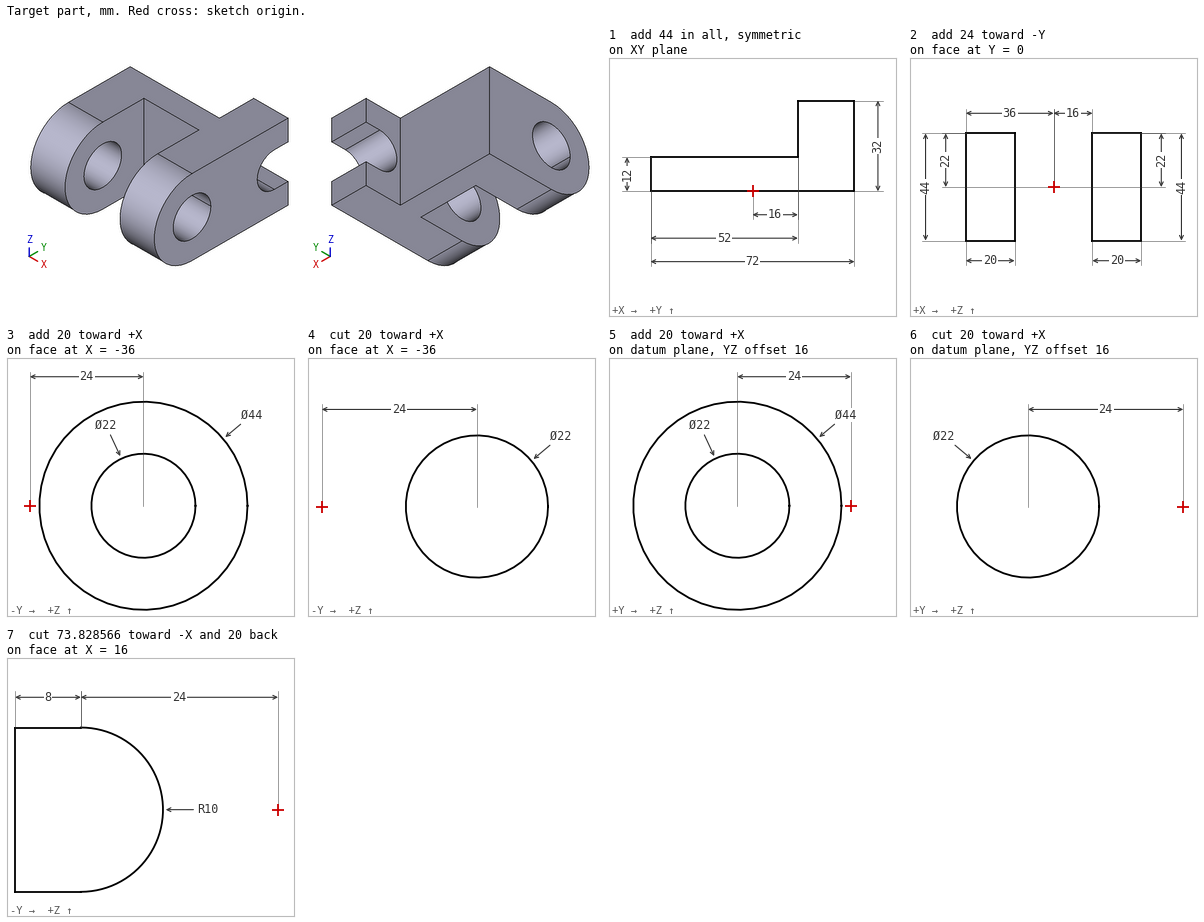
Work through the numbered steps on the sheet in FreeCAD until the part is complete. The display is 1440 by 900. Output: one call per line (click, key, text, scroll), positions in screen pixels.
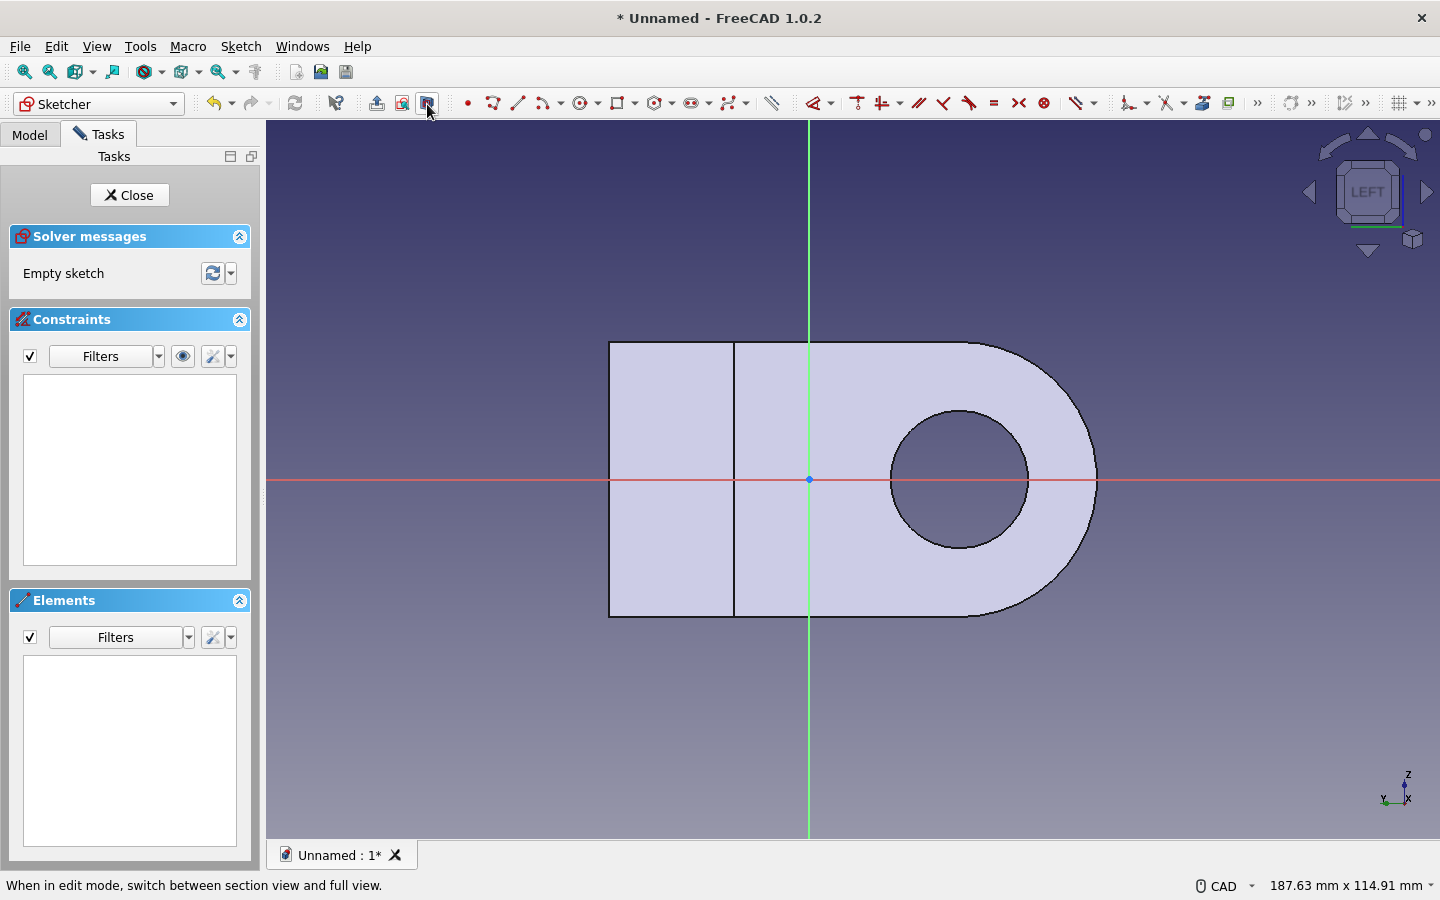
scroll(677, 480, up, 6)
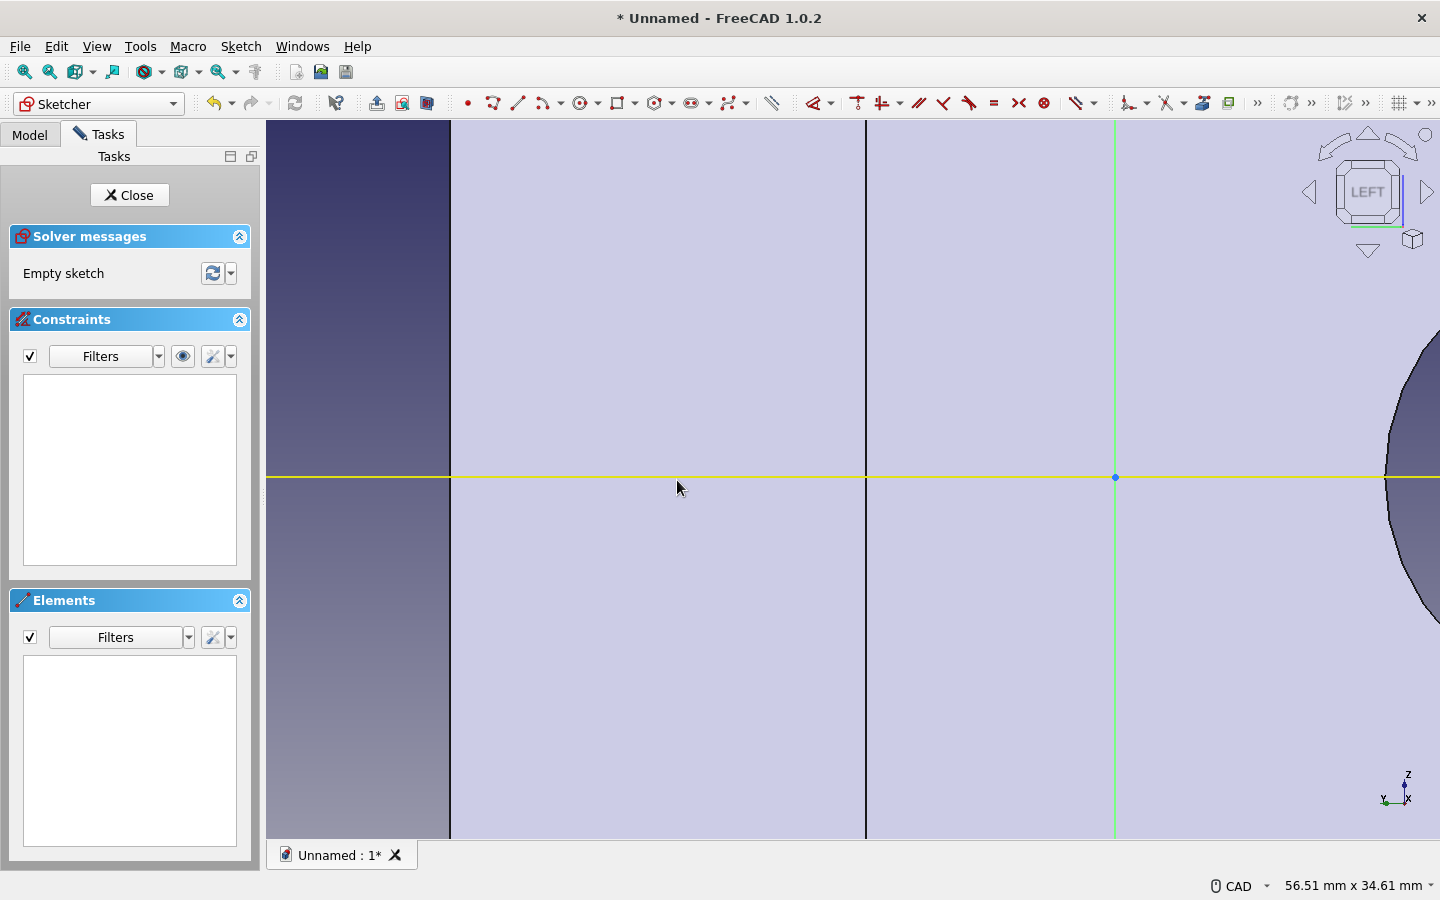
click(493, 104)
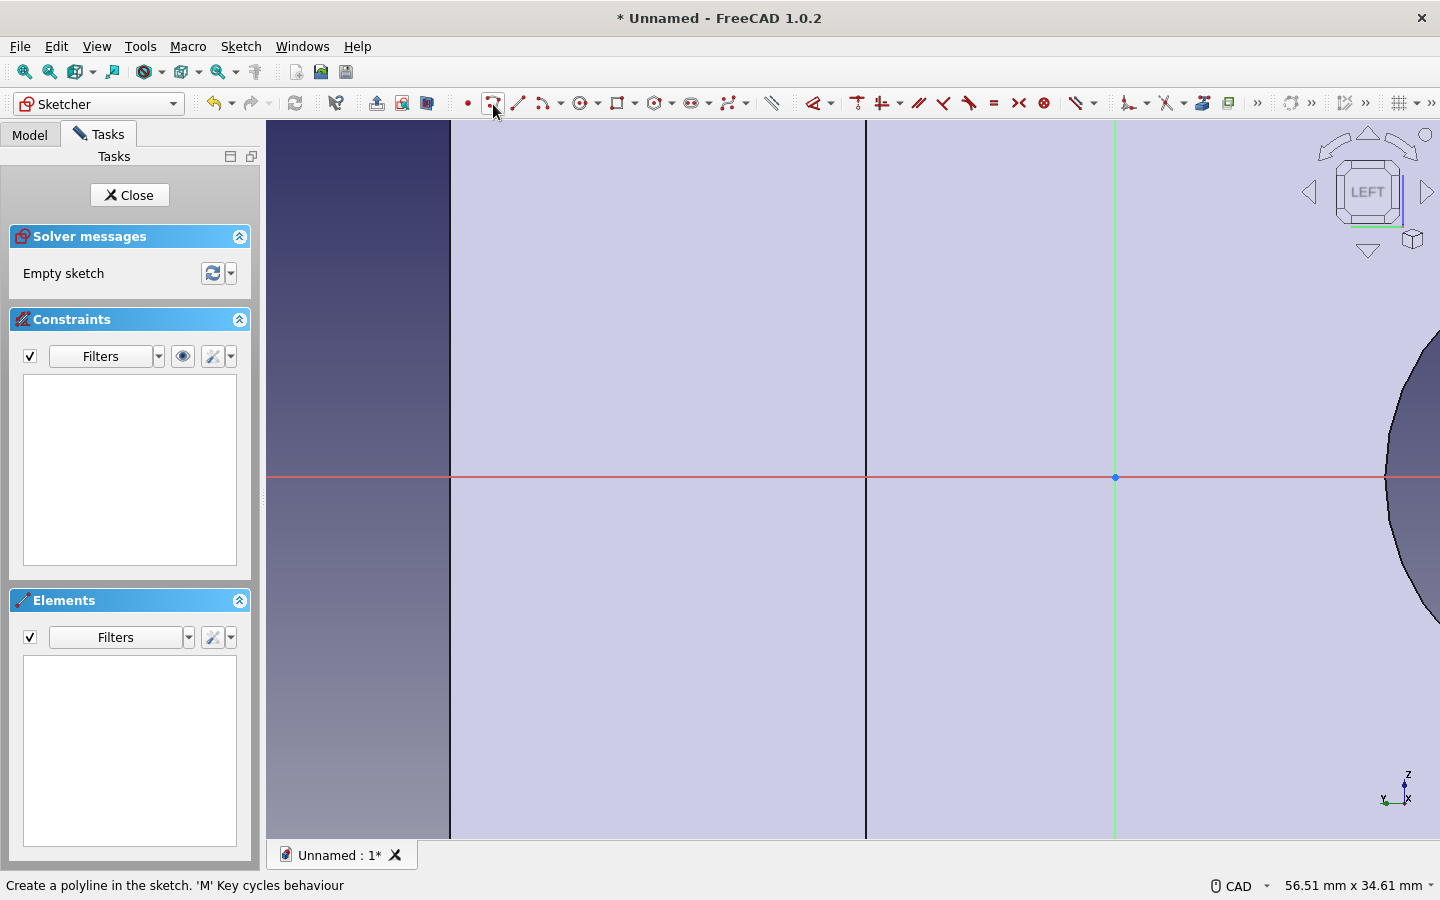
click(617, 269)
click(450, 269)
click(450, 685)
click(617, 685)
right_click(617, 685)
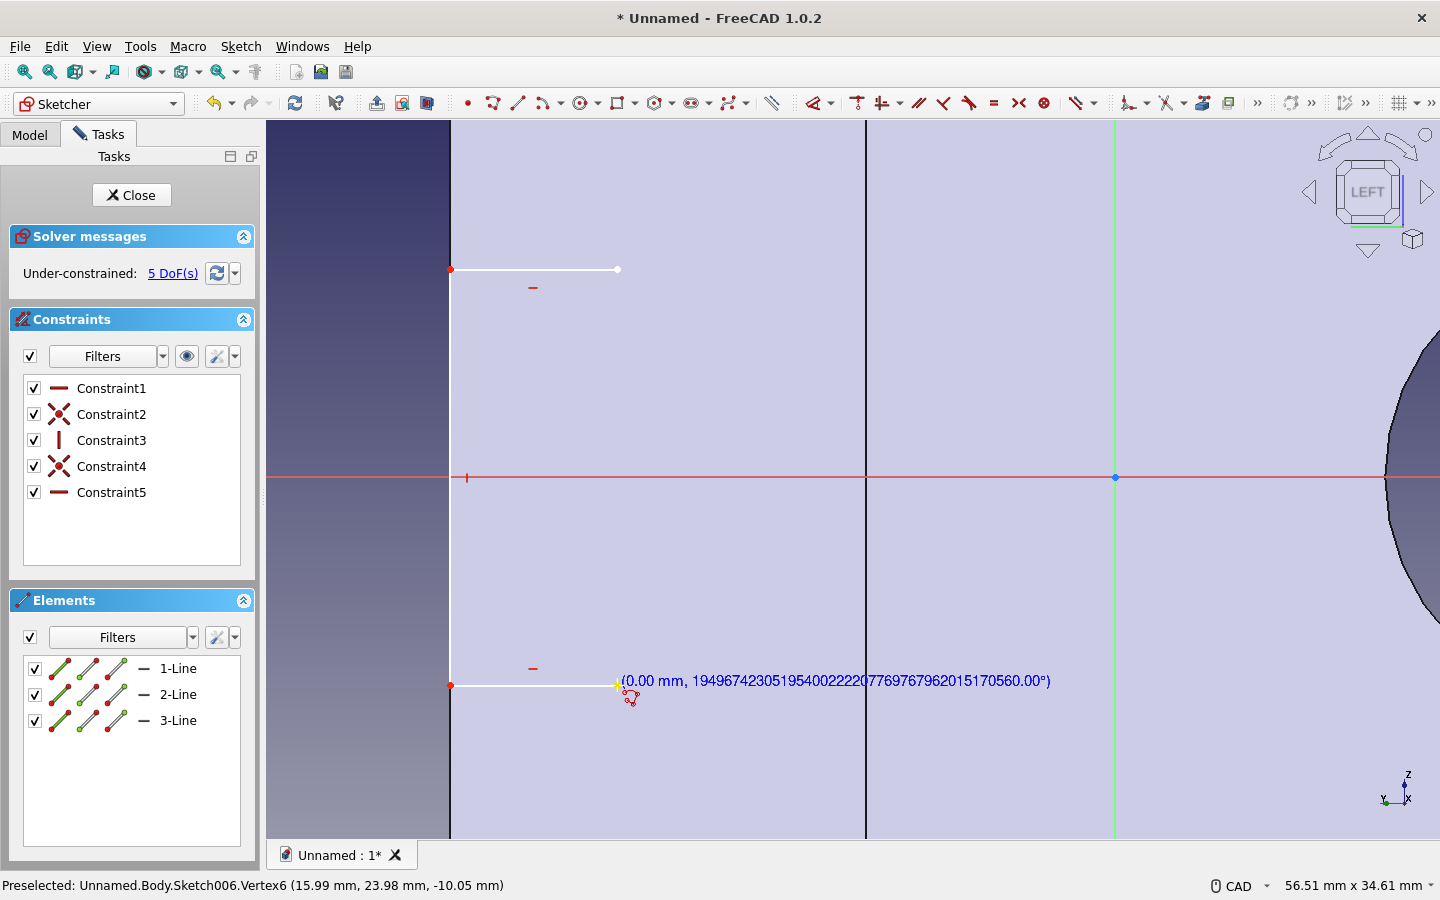
key(g)
key(3)
key(a)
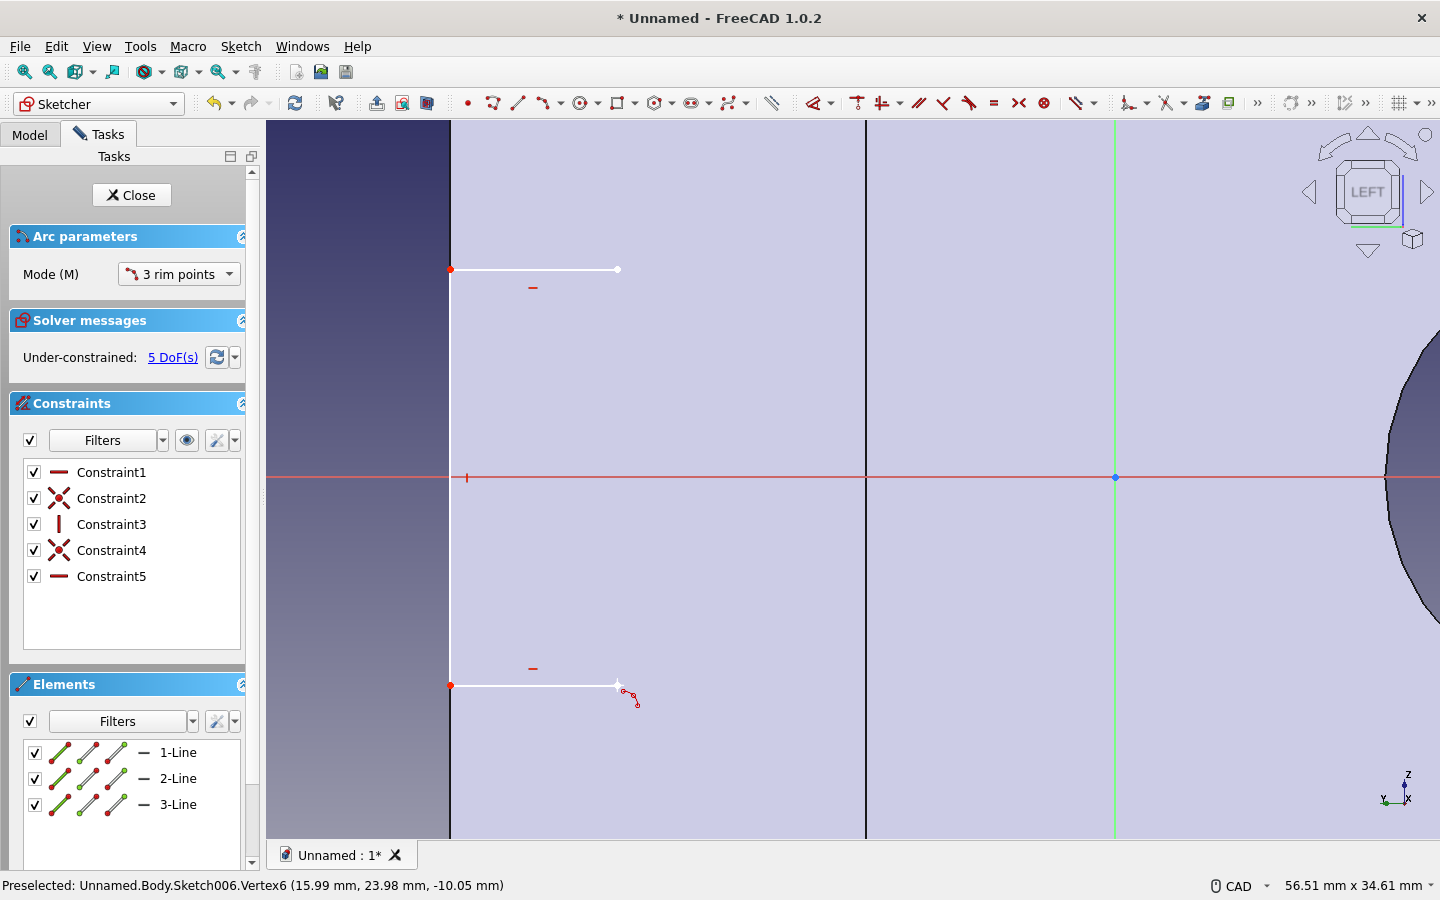
click(617, 686)
click(617, 270)
click(814, 541)
key(Escape)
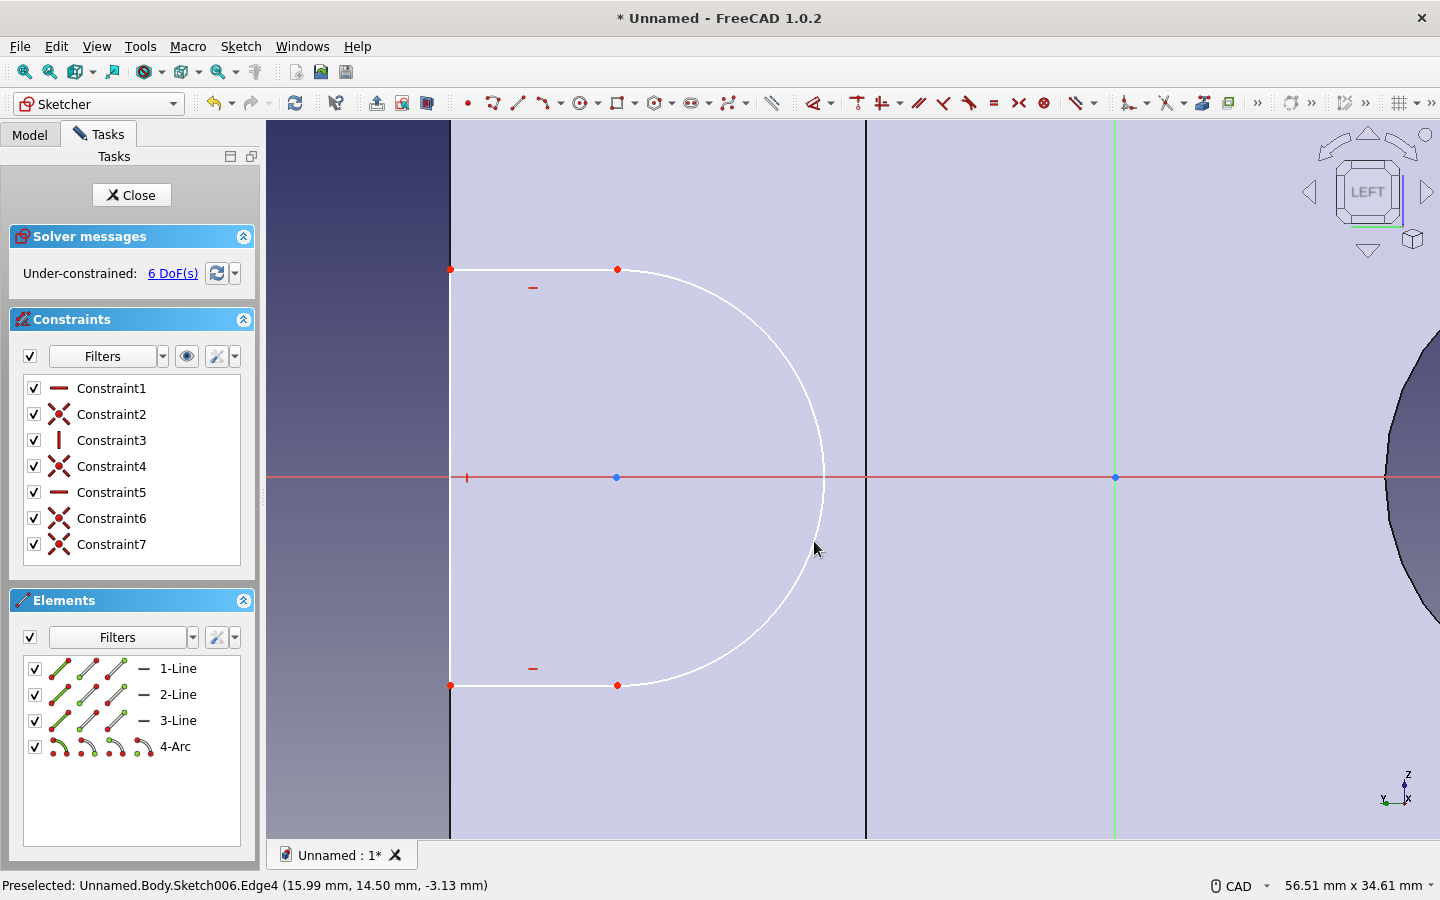
click(567, 270)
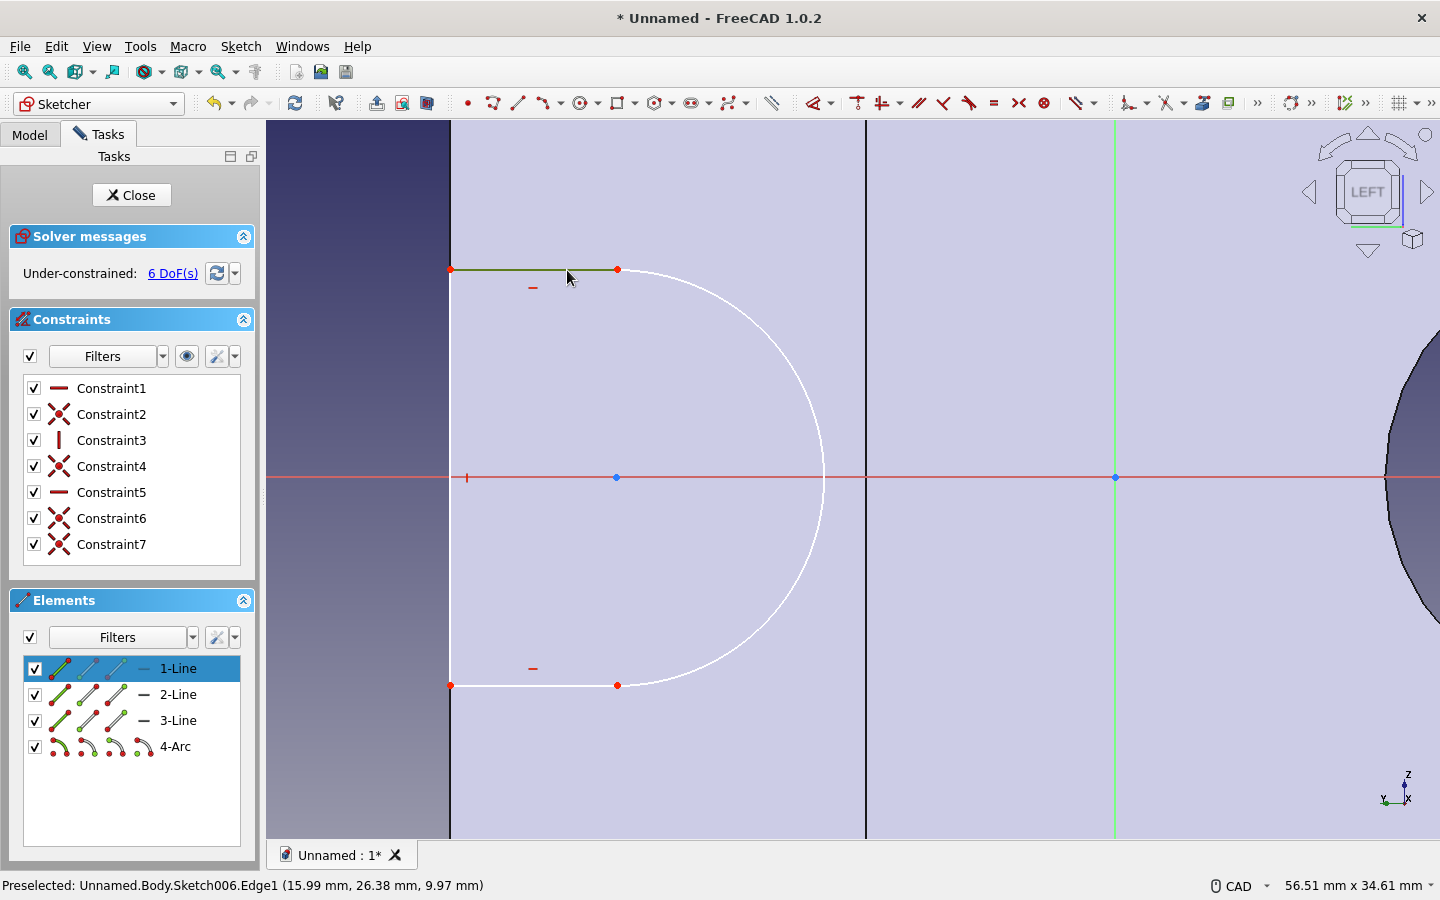
click(785, 600)